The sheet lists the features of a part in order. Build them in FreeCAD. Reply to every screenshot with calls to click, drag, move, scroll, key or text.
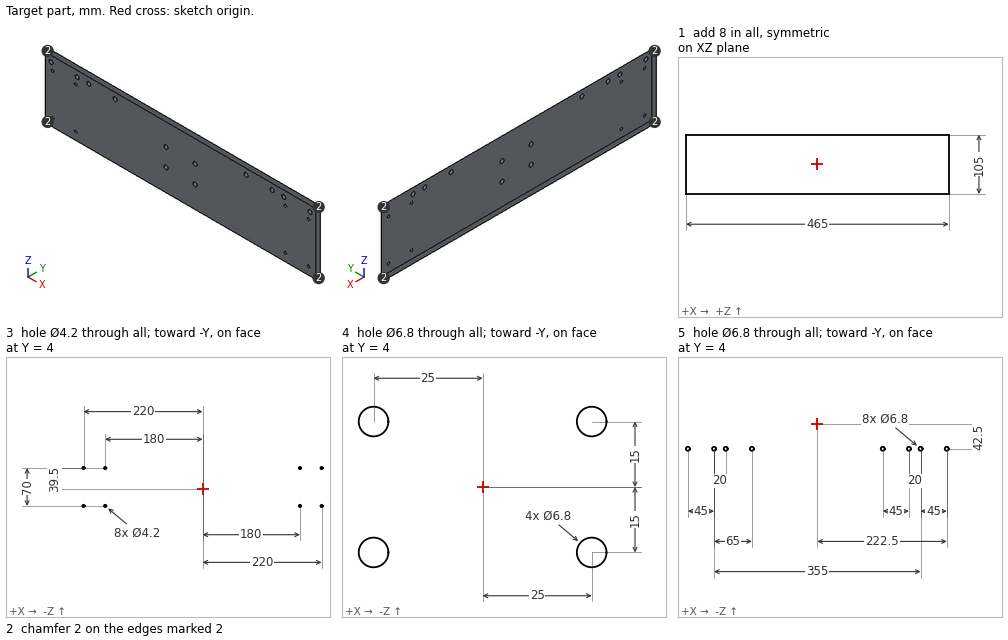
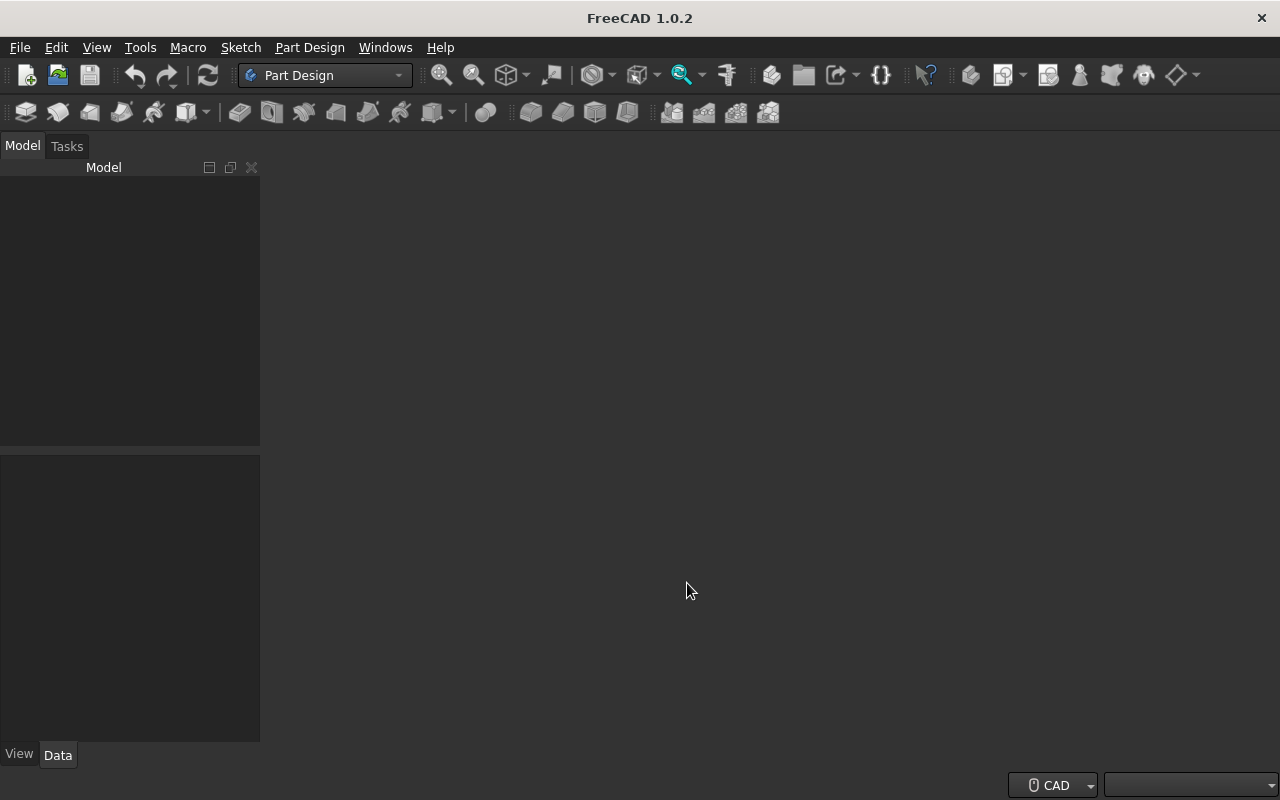
click(26, 76)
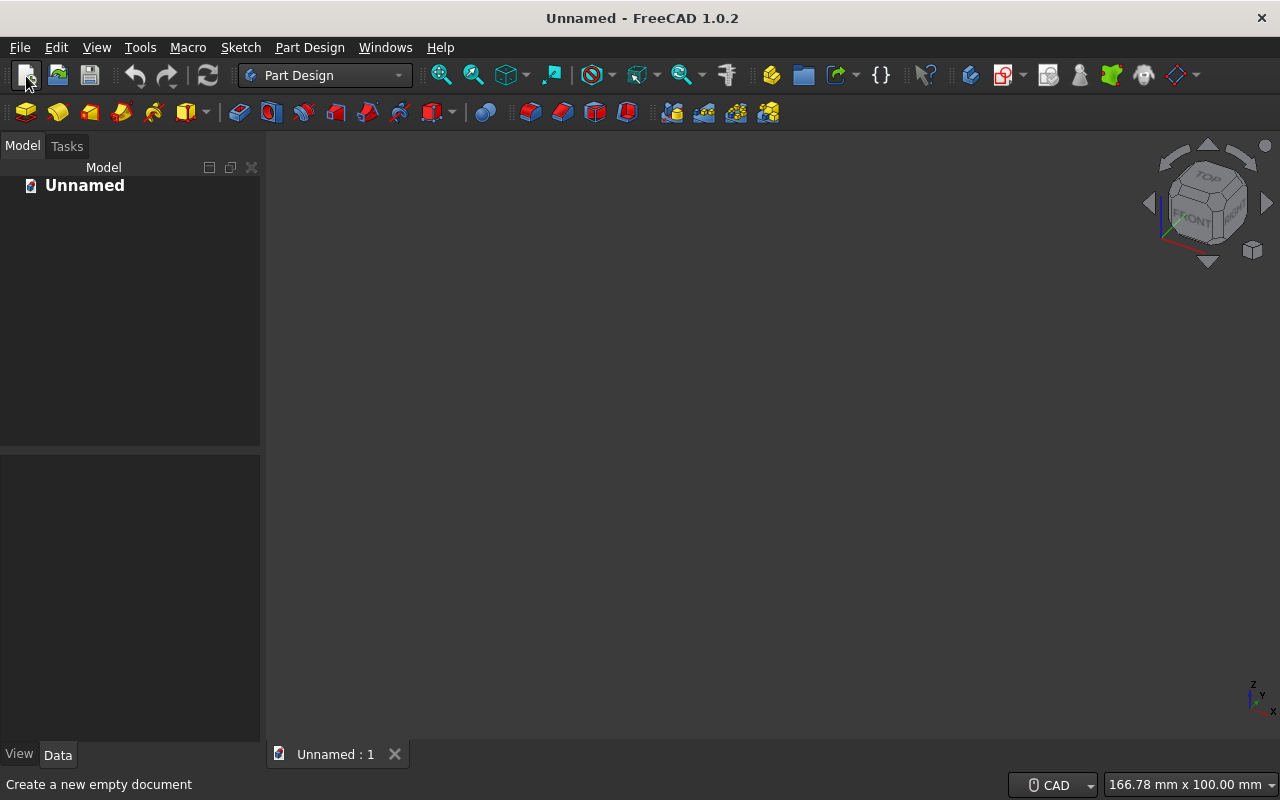
click(1004, 76)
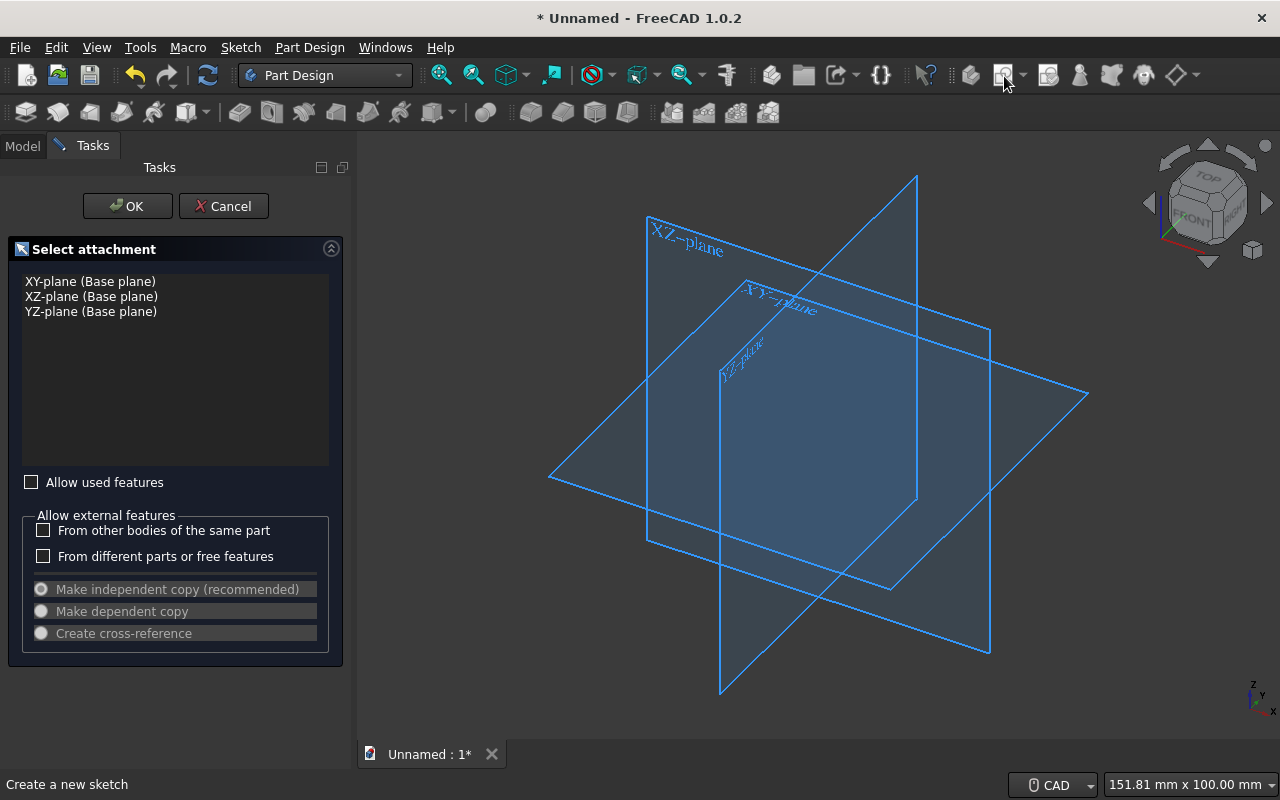
click(82, 296)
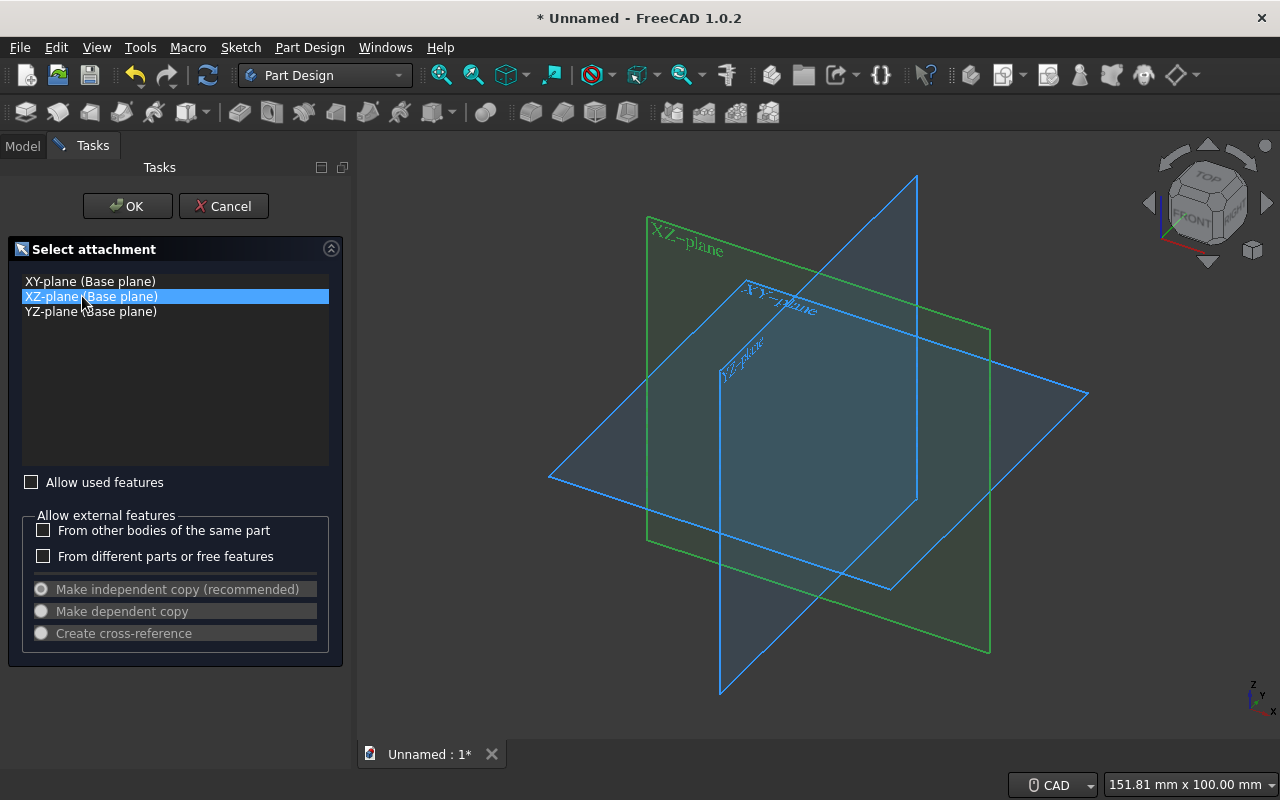
click(128, 206)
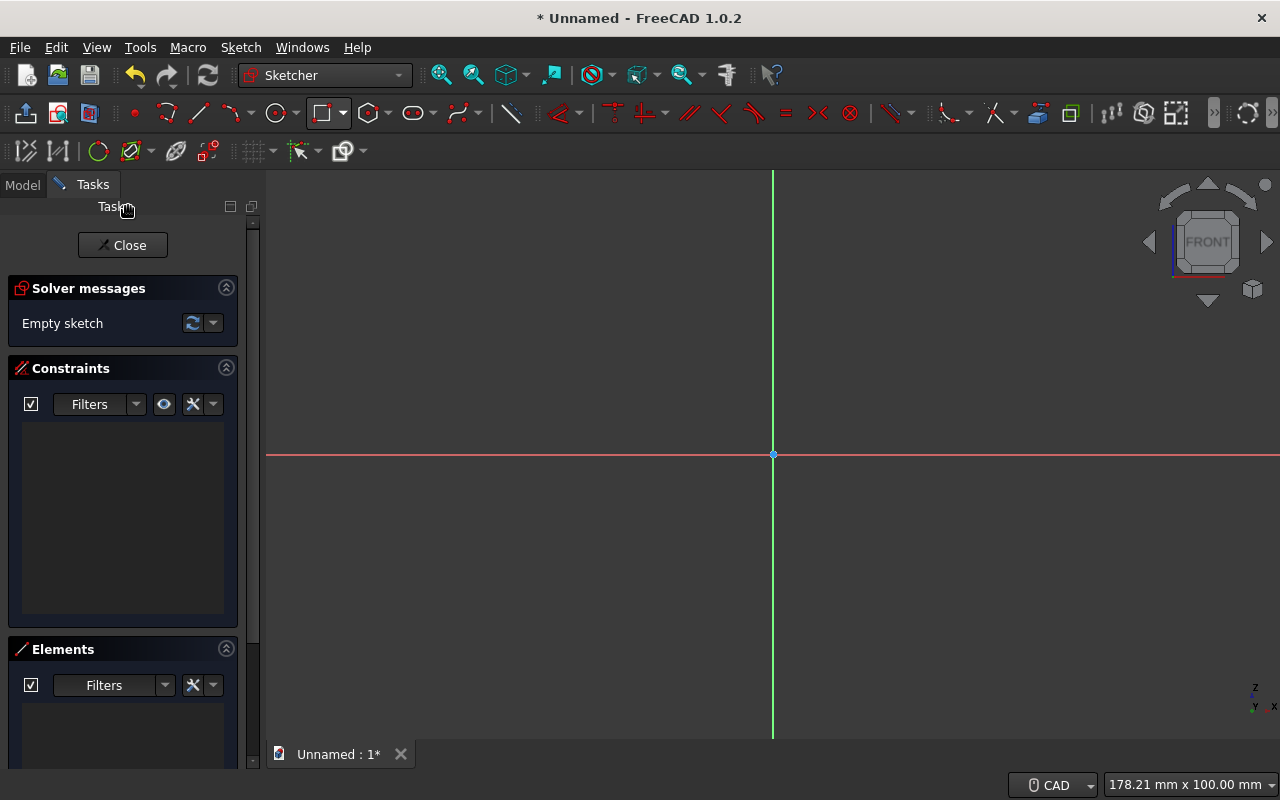
scroll(687, 454, down, 8)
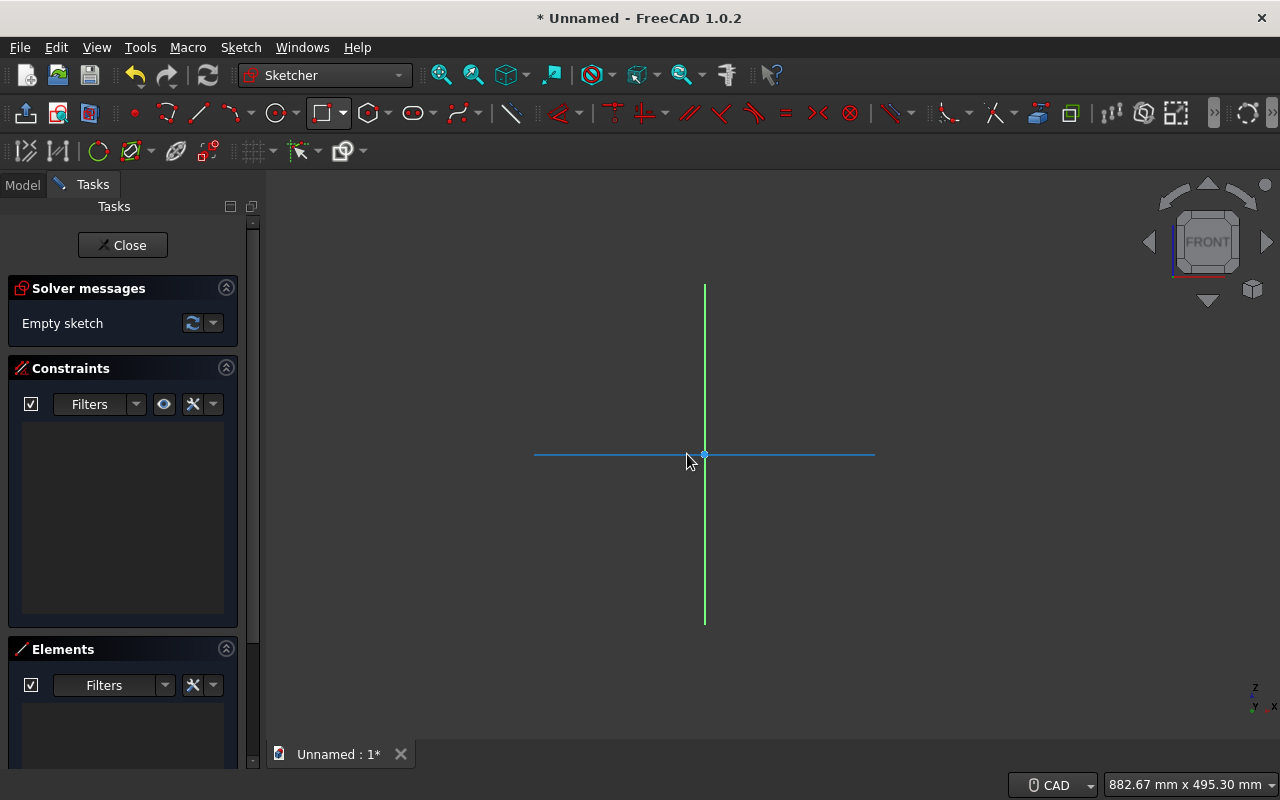
click(346, 114)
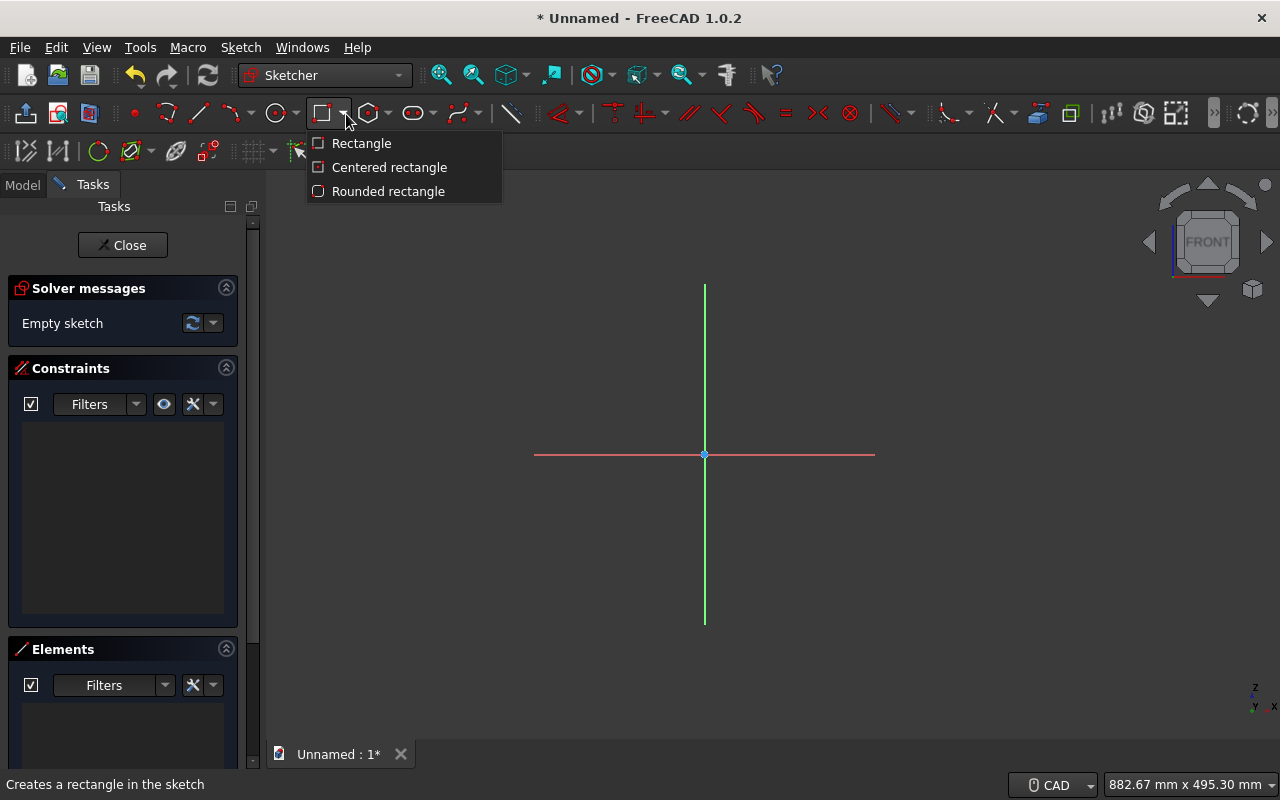
click(404, 167)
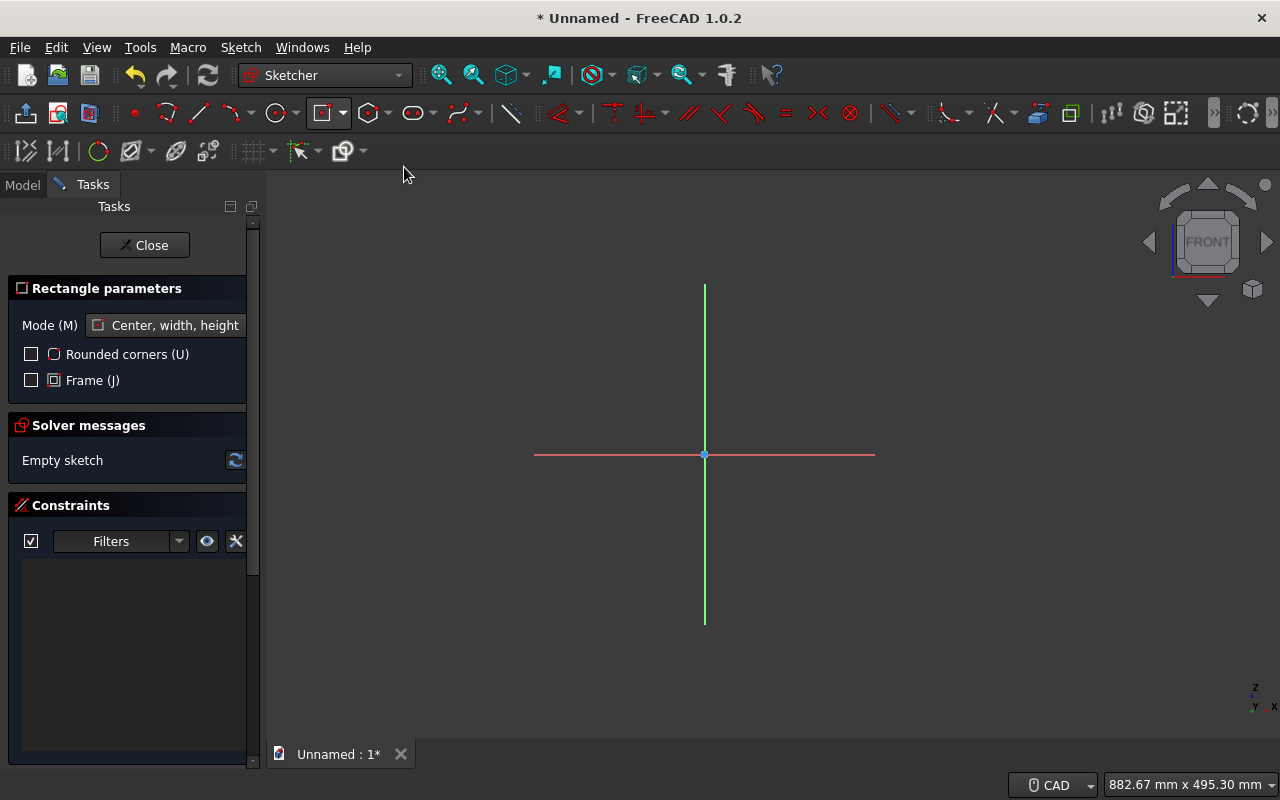
click(705, 454)
move(972, 394)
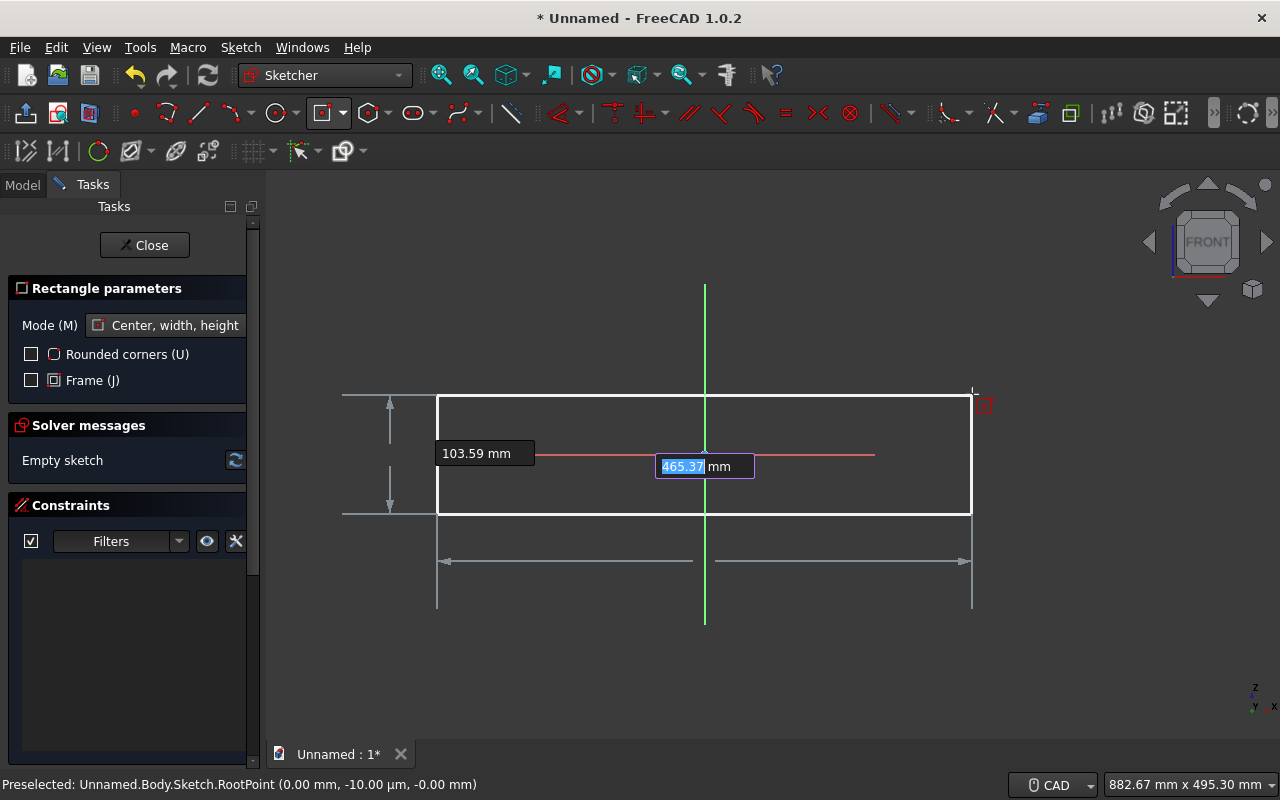
text(465)
key(Tab)
text(105)
key(Return)
key(Escape)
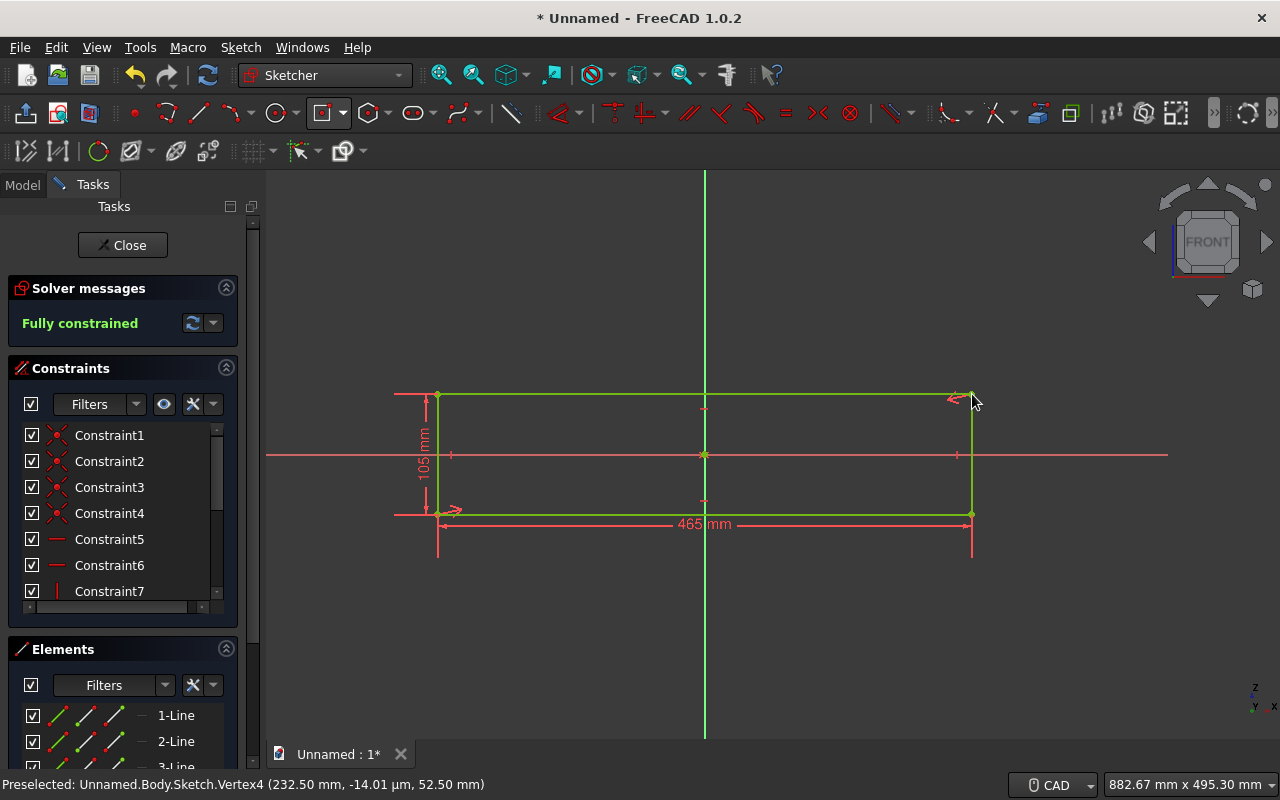
click(123, 245)